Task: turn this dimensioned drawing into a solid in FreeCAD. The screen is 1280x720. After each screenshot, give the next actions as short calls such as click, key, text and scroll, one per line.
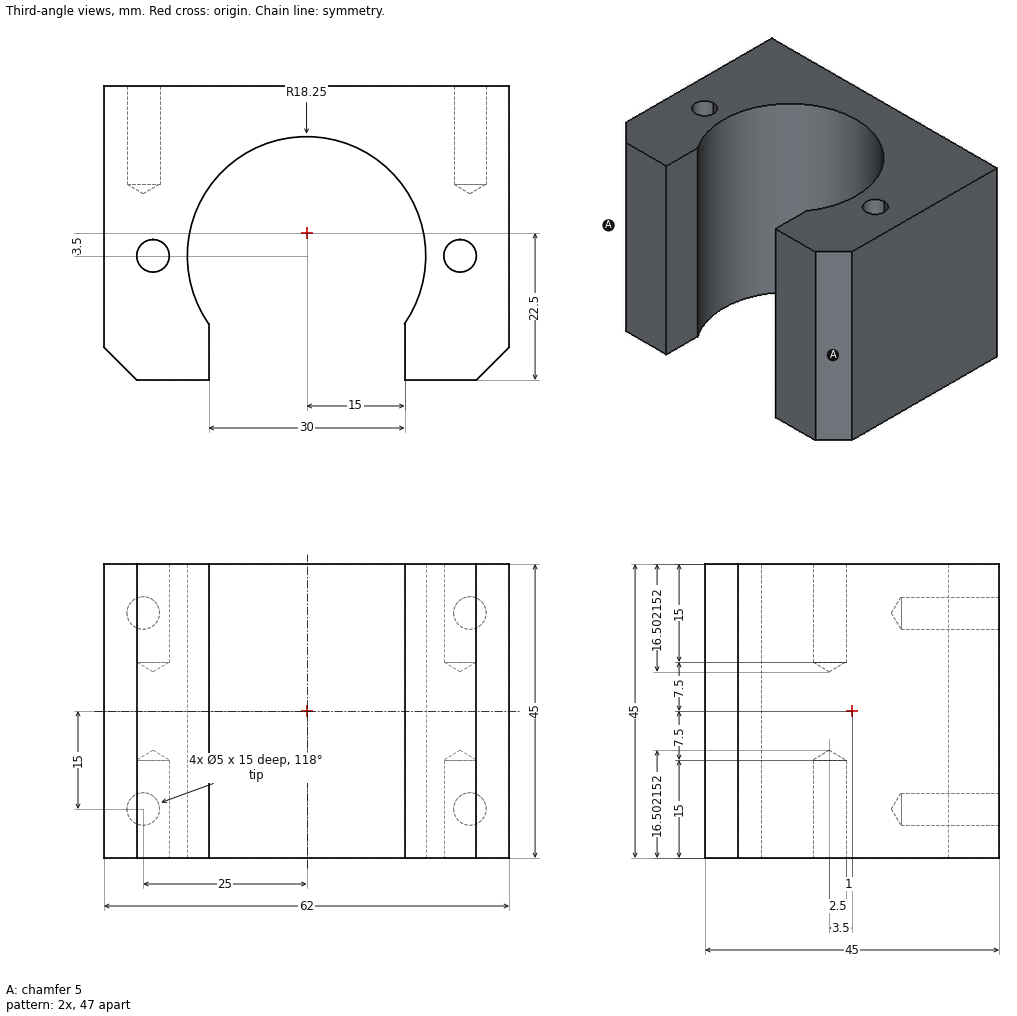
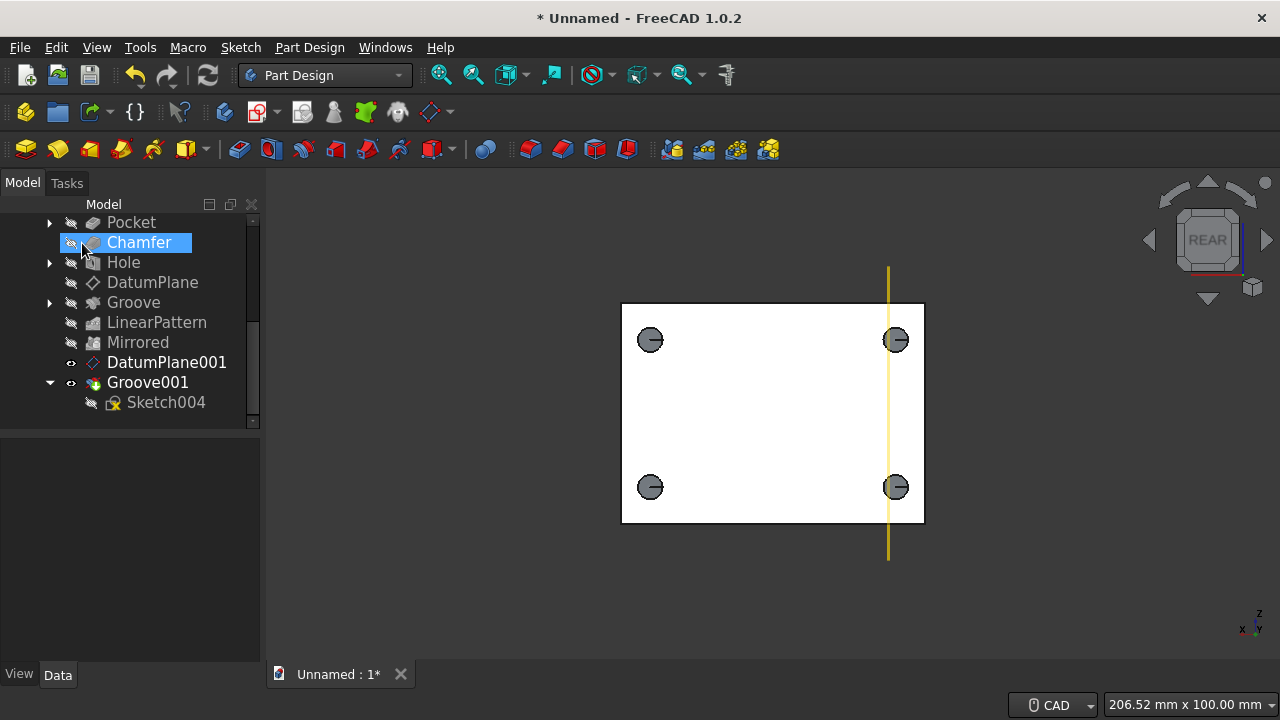
click(116, 363)
key(space)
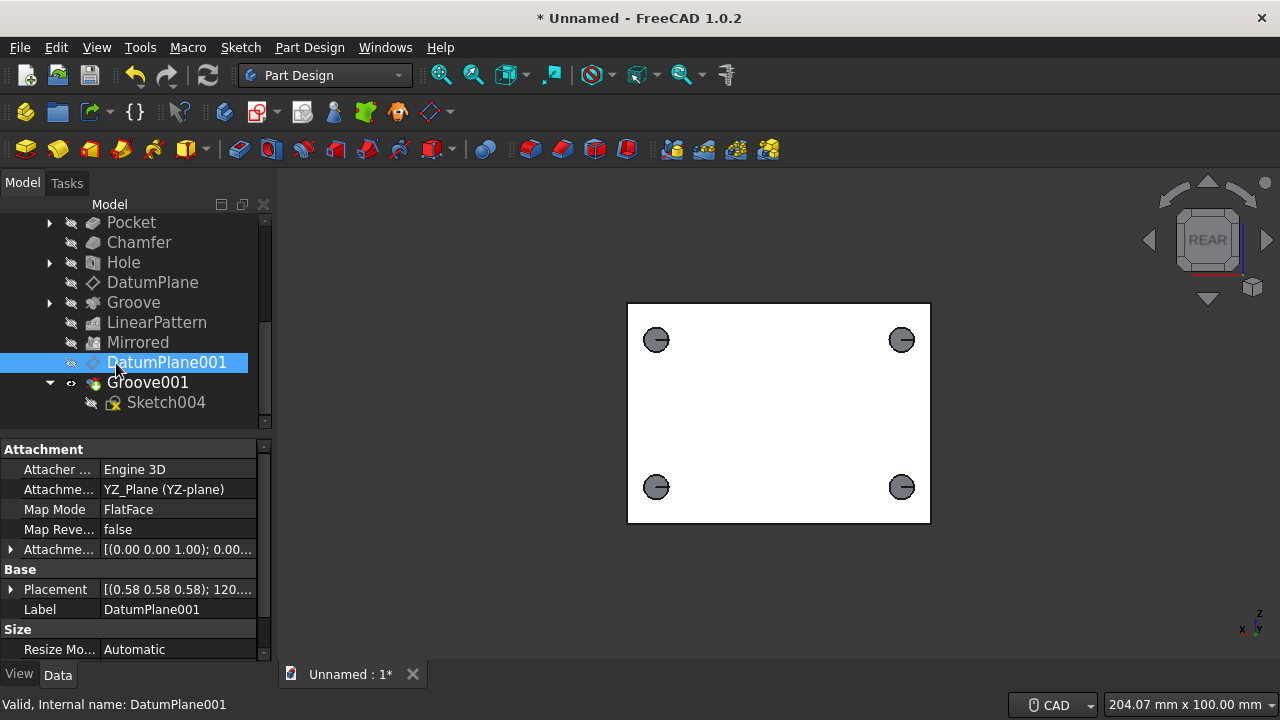
key(0)